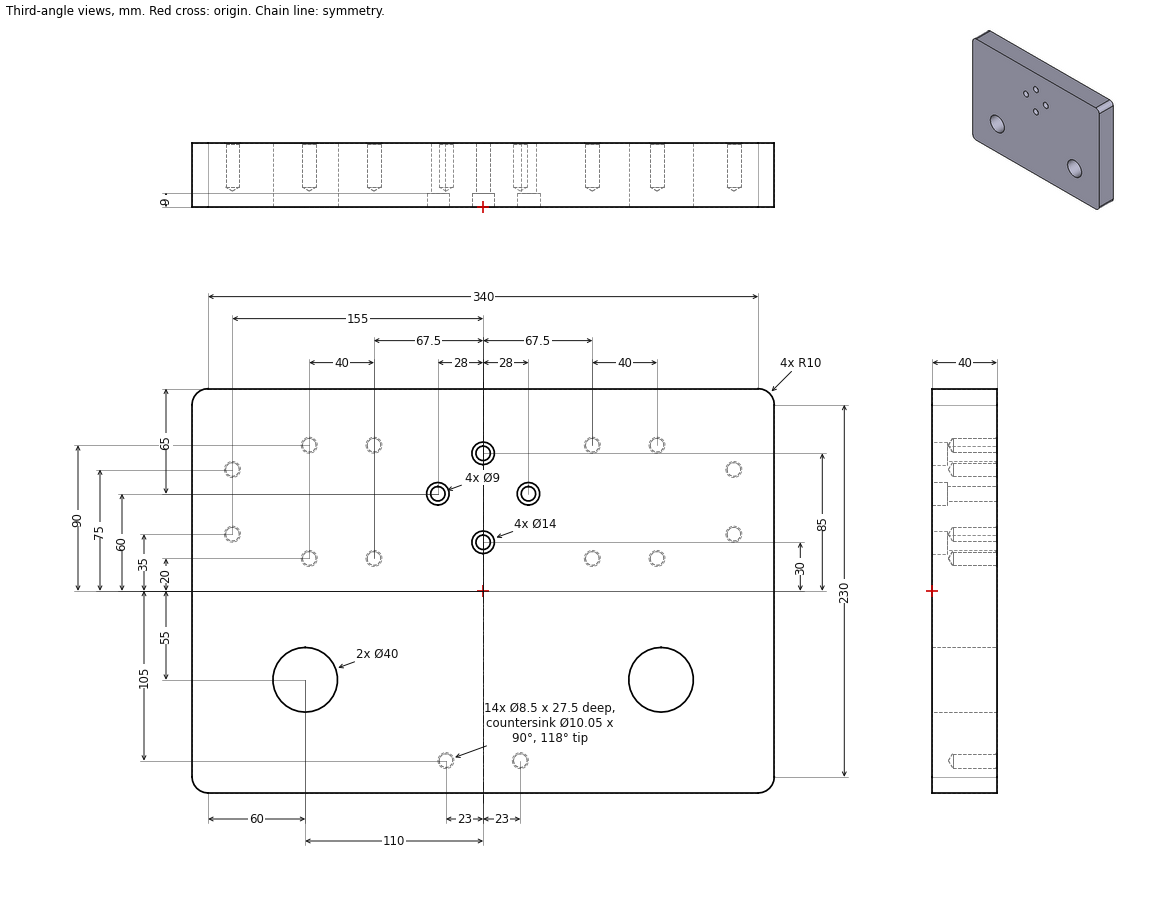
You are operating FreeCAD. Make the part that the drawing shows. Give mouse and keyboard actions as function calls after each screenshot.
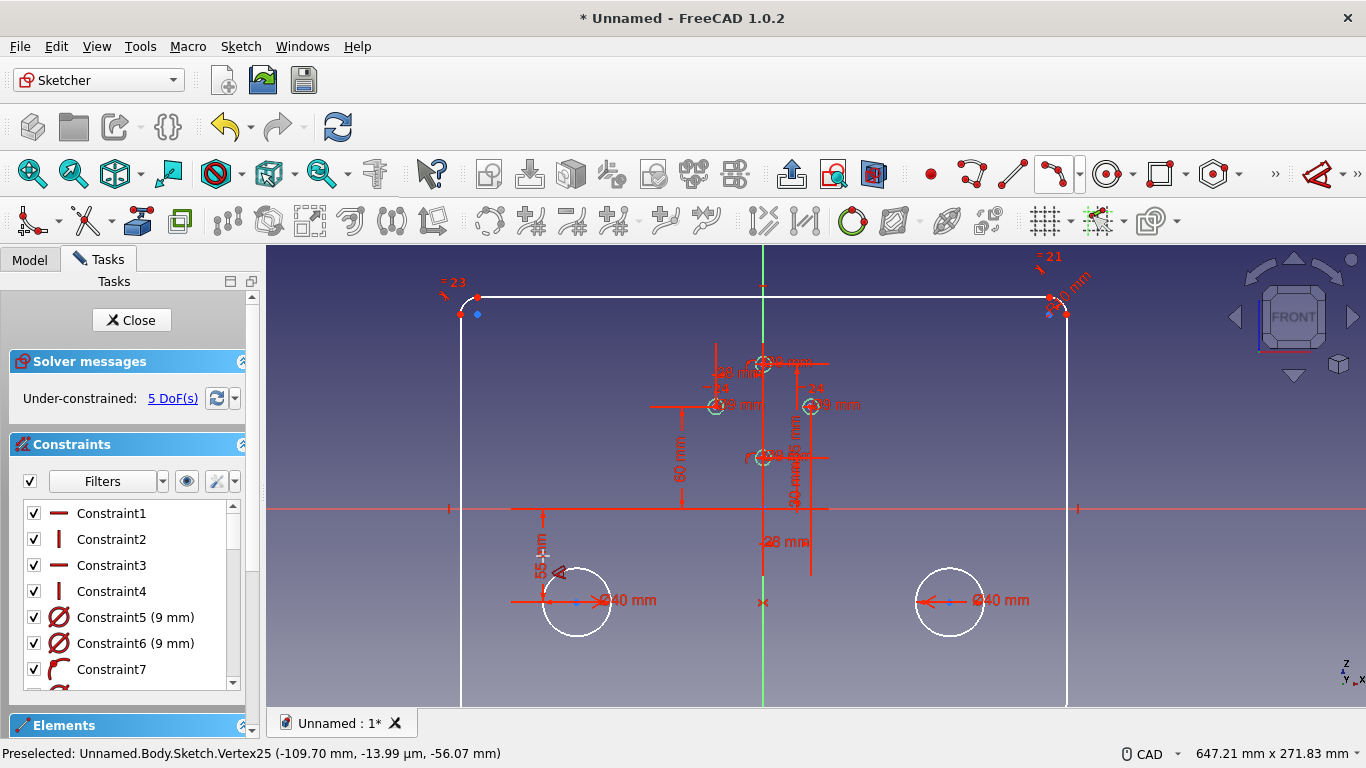
click(649, 297)
click(632, 331)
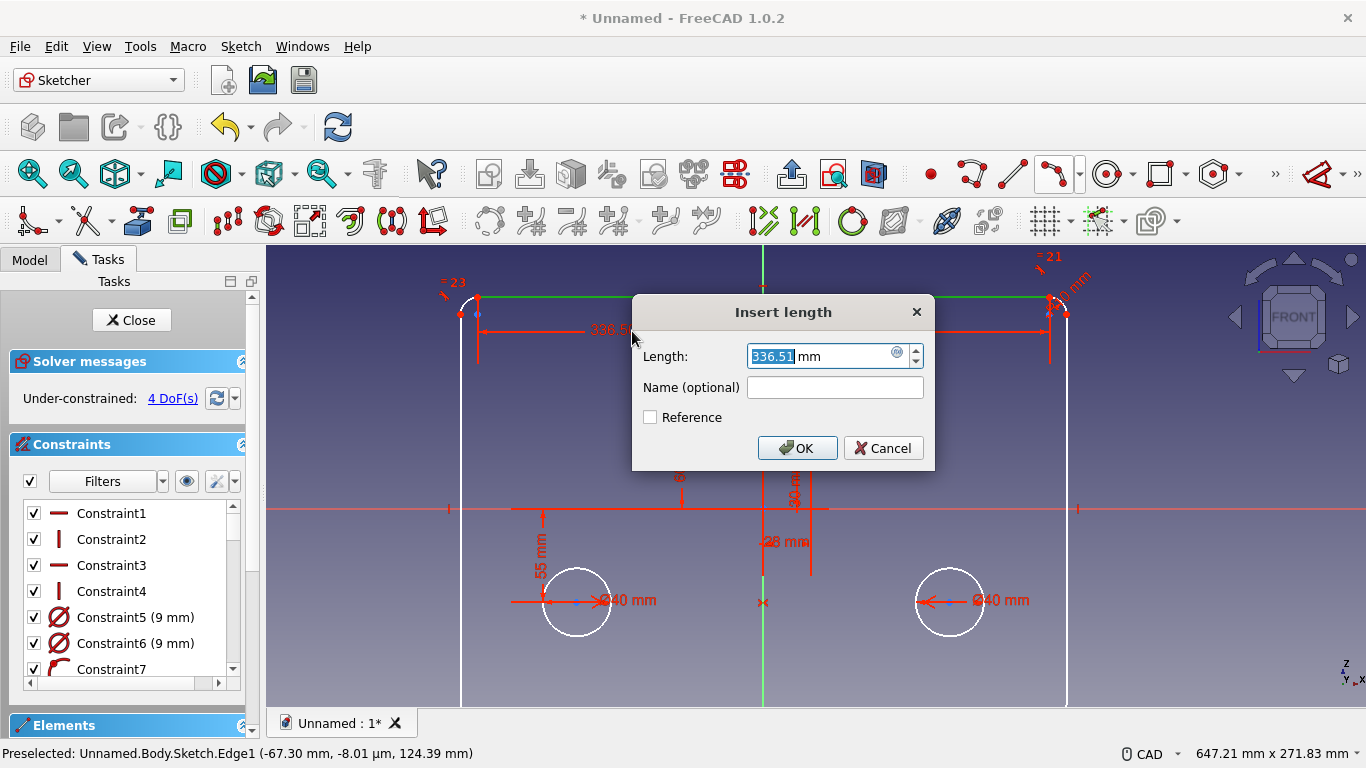
text(340)
key(Return)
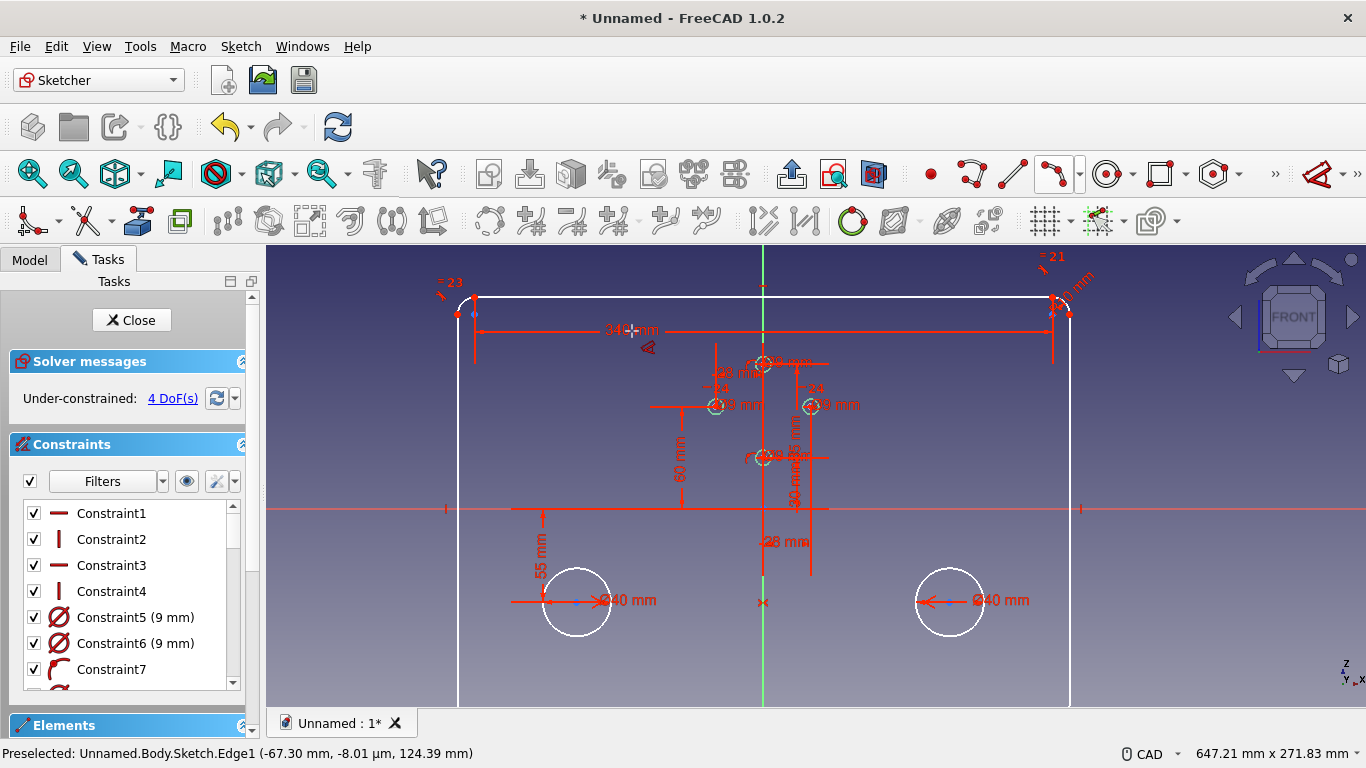
click(1070, 431)
click(1104, 413)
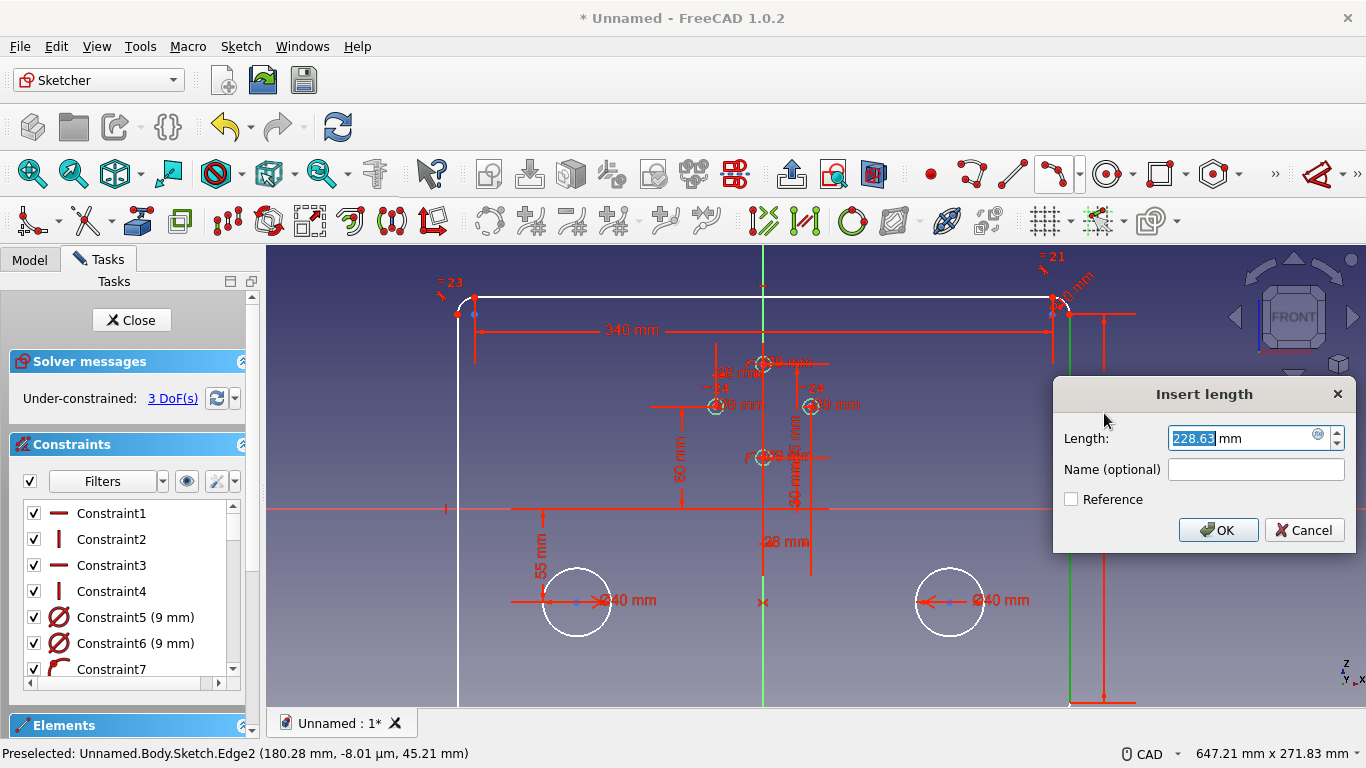
text(230)
key(Return)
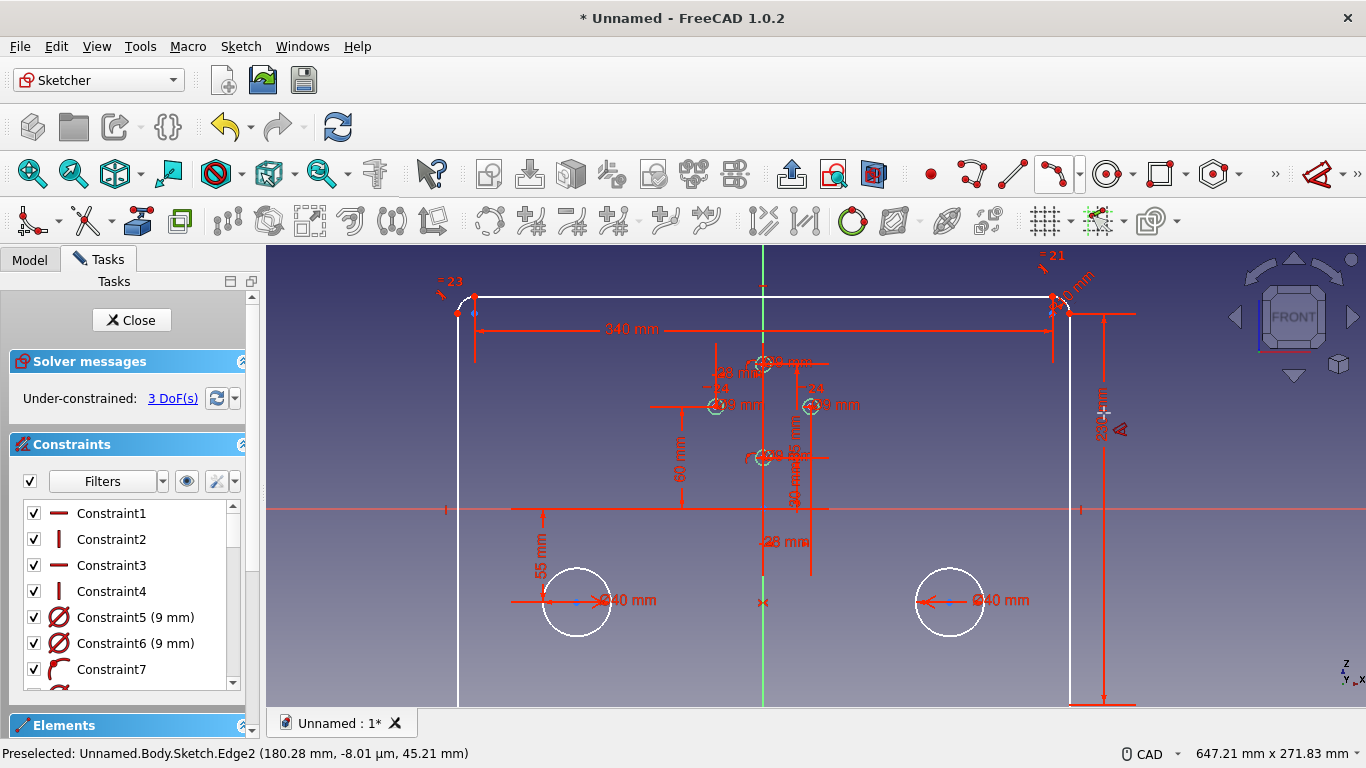
click(577, 602)
click(670, 636)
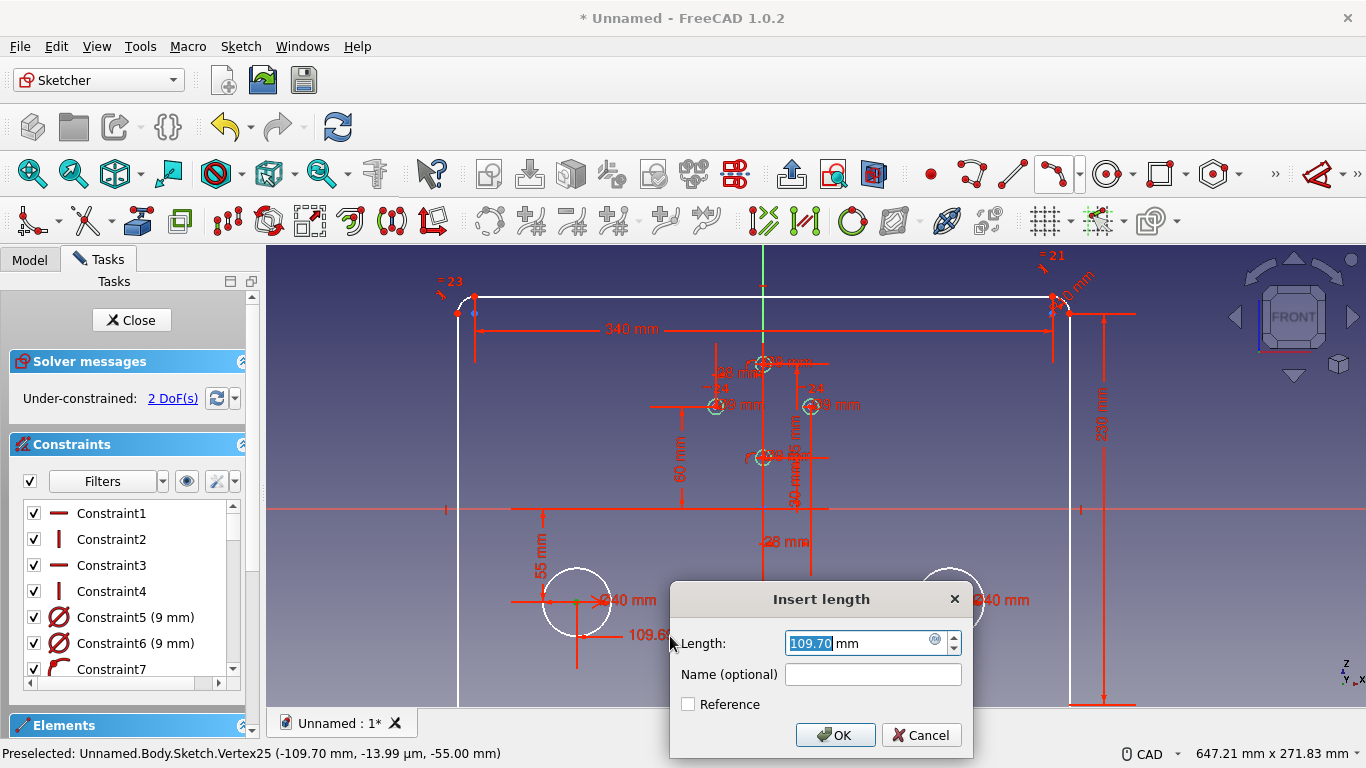
text(110)
key(Return)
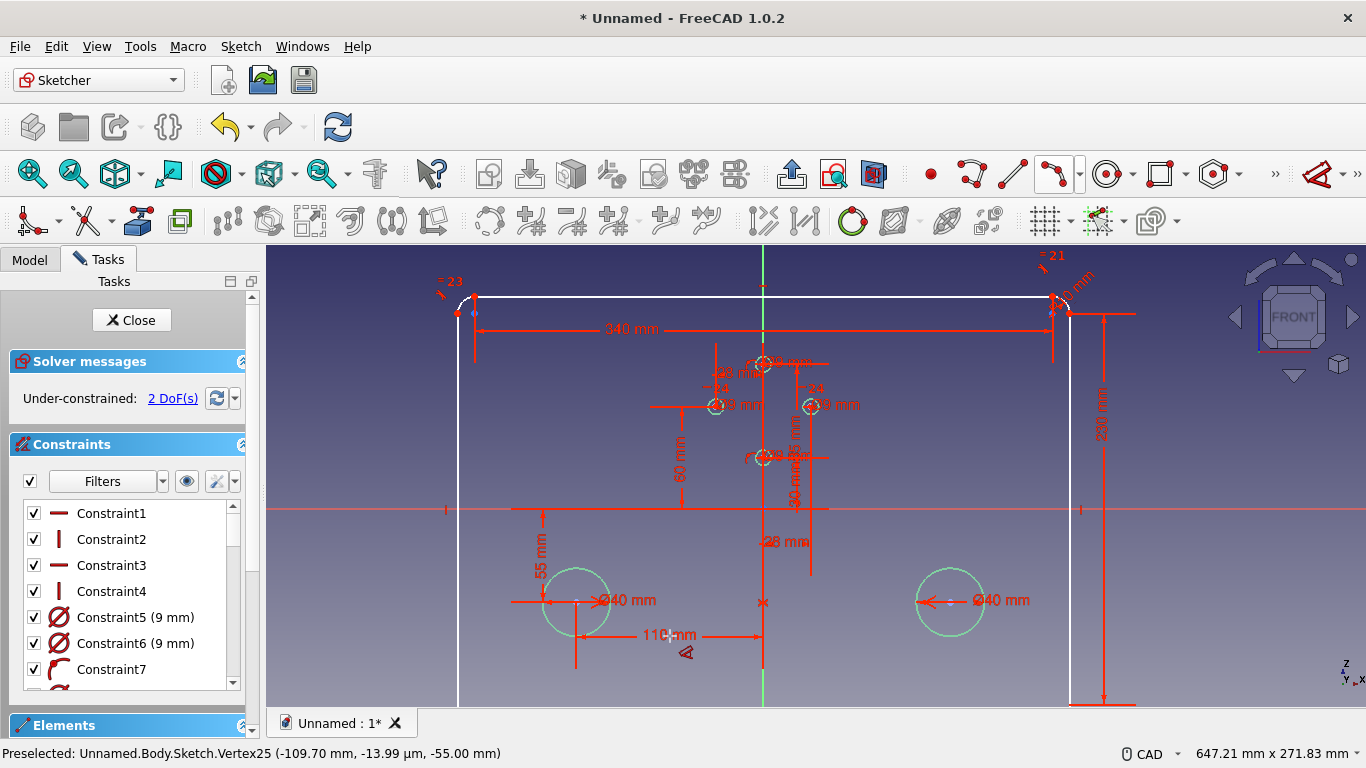
click(475, 297)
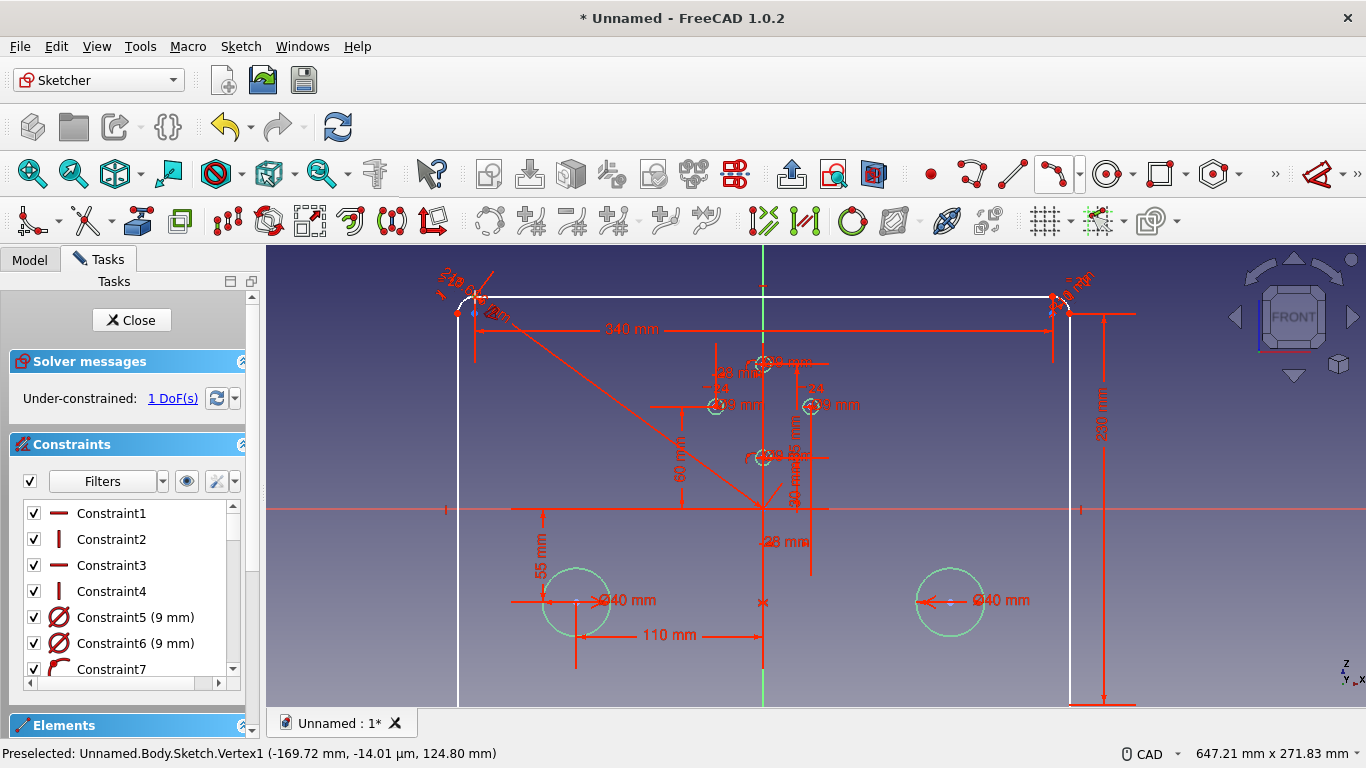
click(716, 407)
click(441, 352)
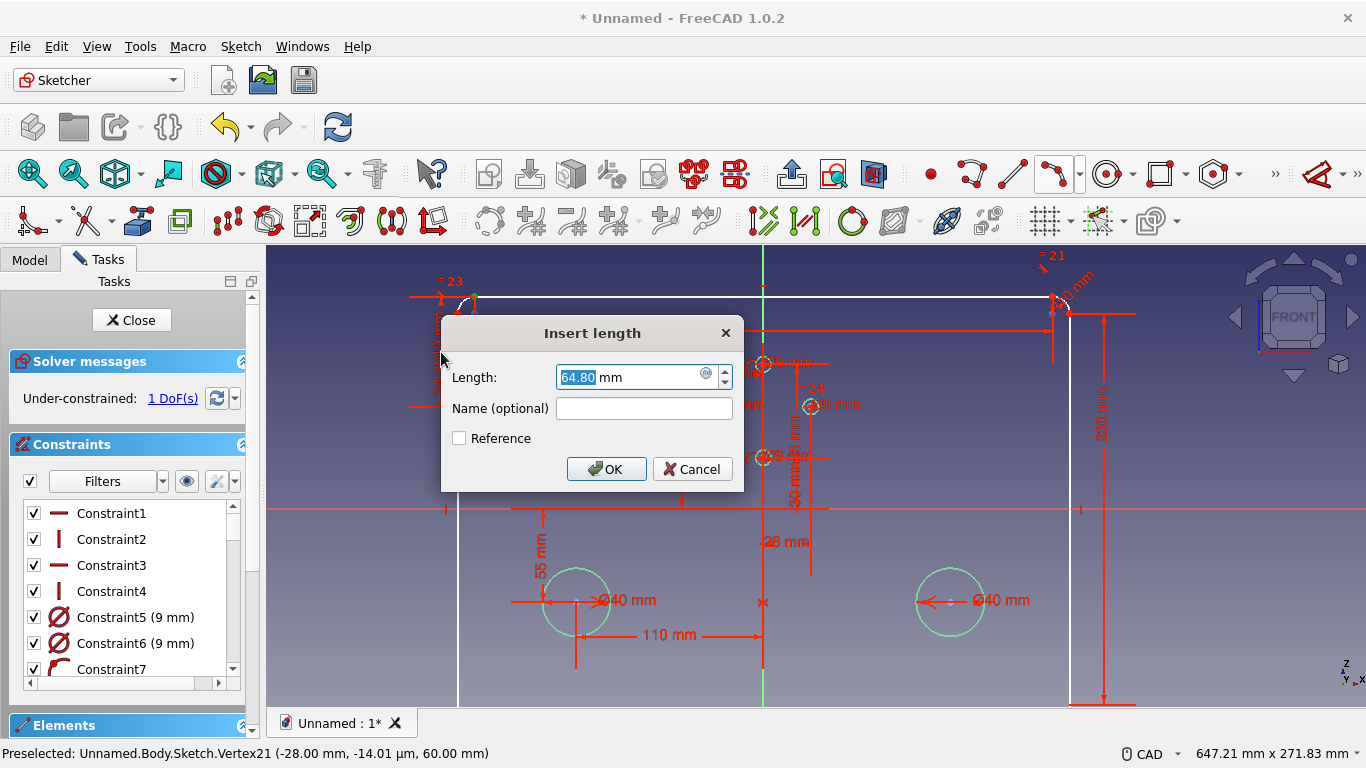
text(65)
key(Return)